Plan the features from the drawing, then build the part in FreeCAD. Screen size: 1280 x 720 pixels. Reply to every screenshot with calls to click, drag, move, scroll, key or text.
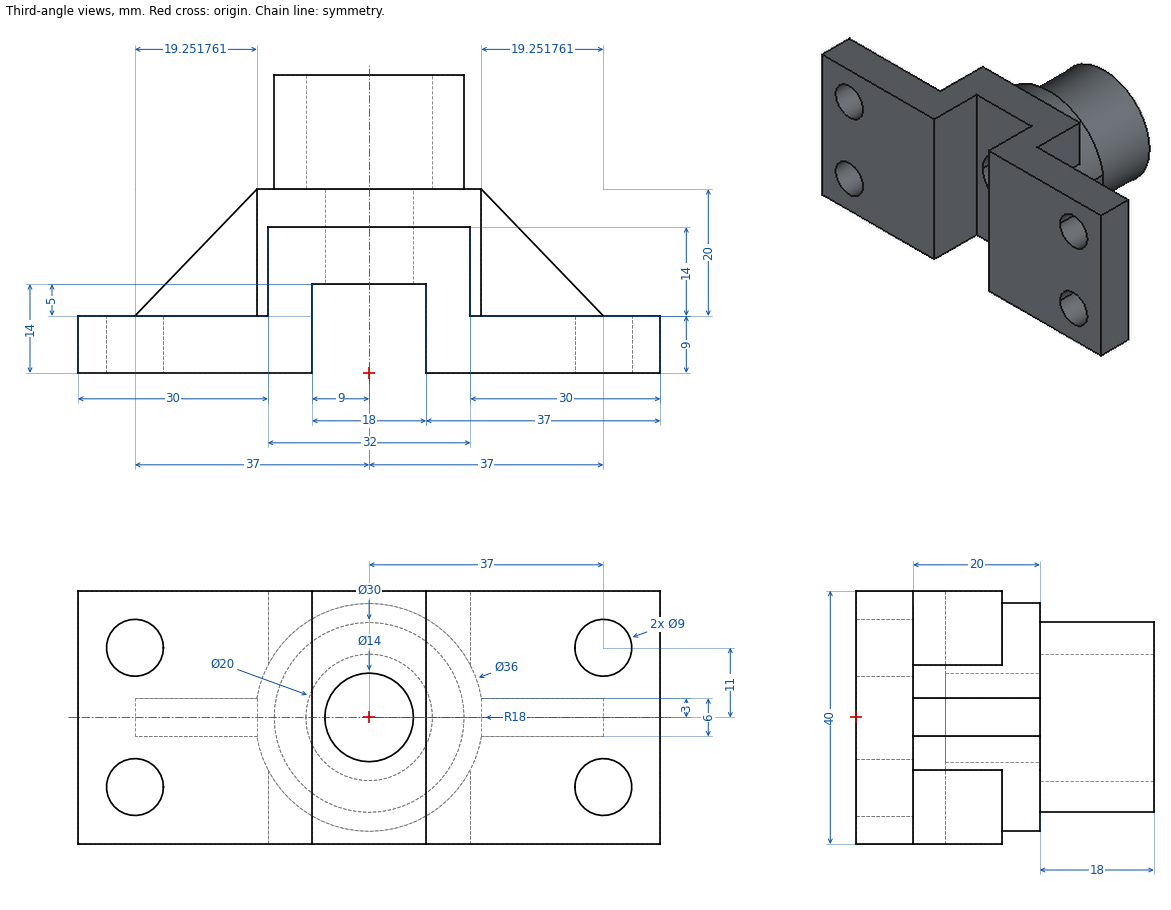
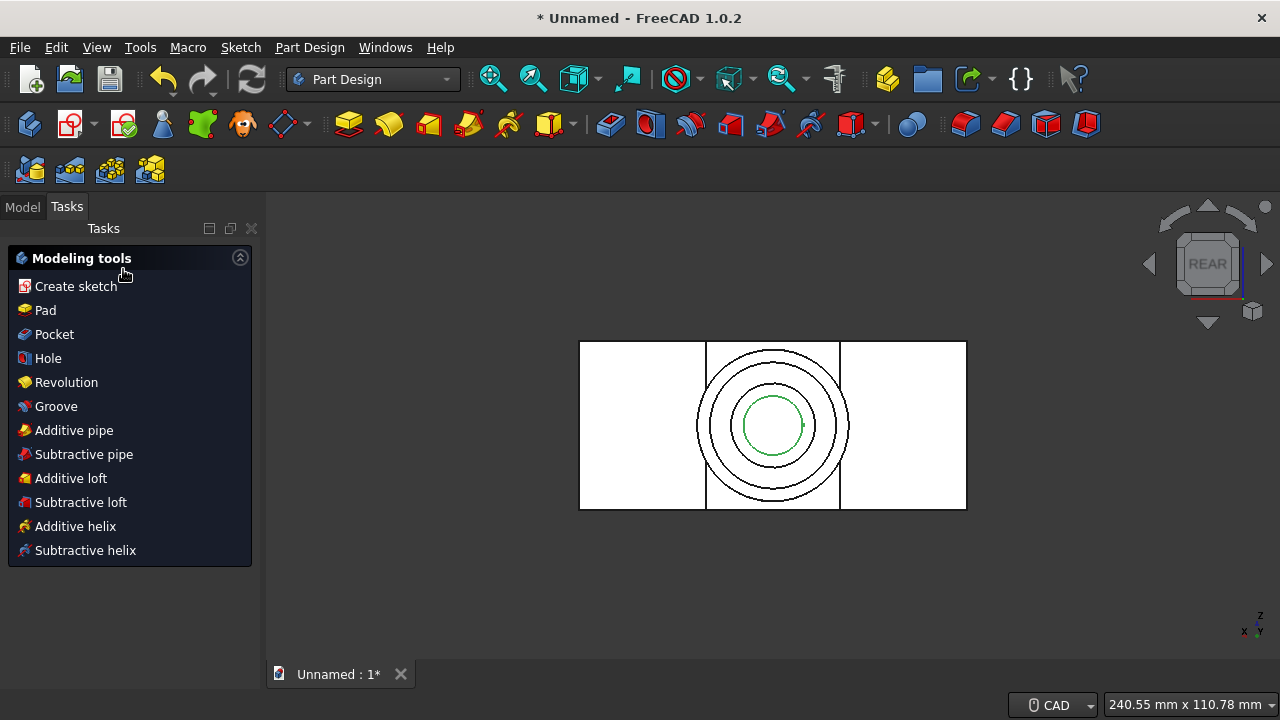
click(612, 124)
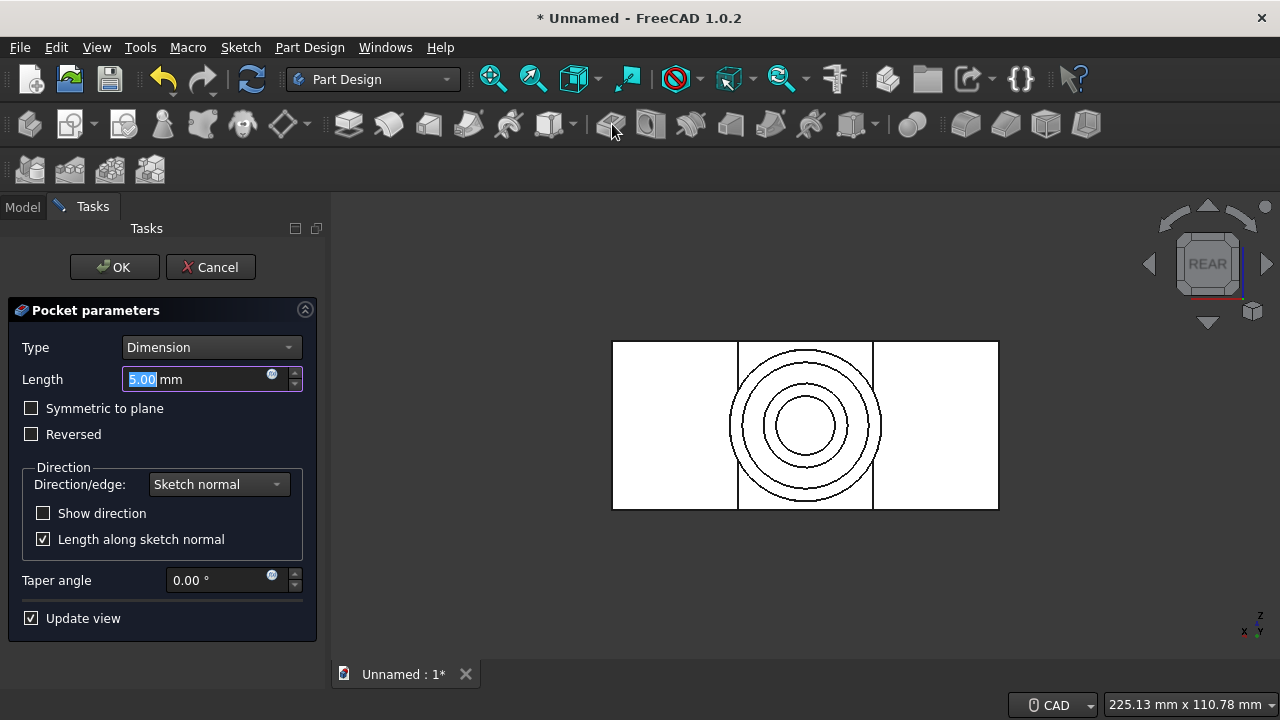
click(212, 348)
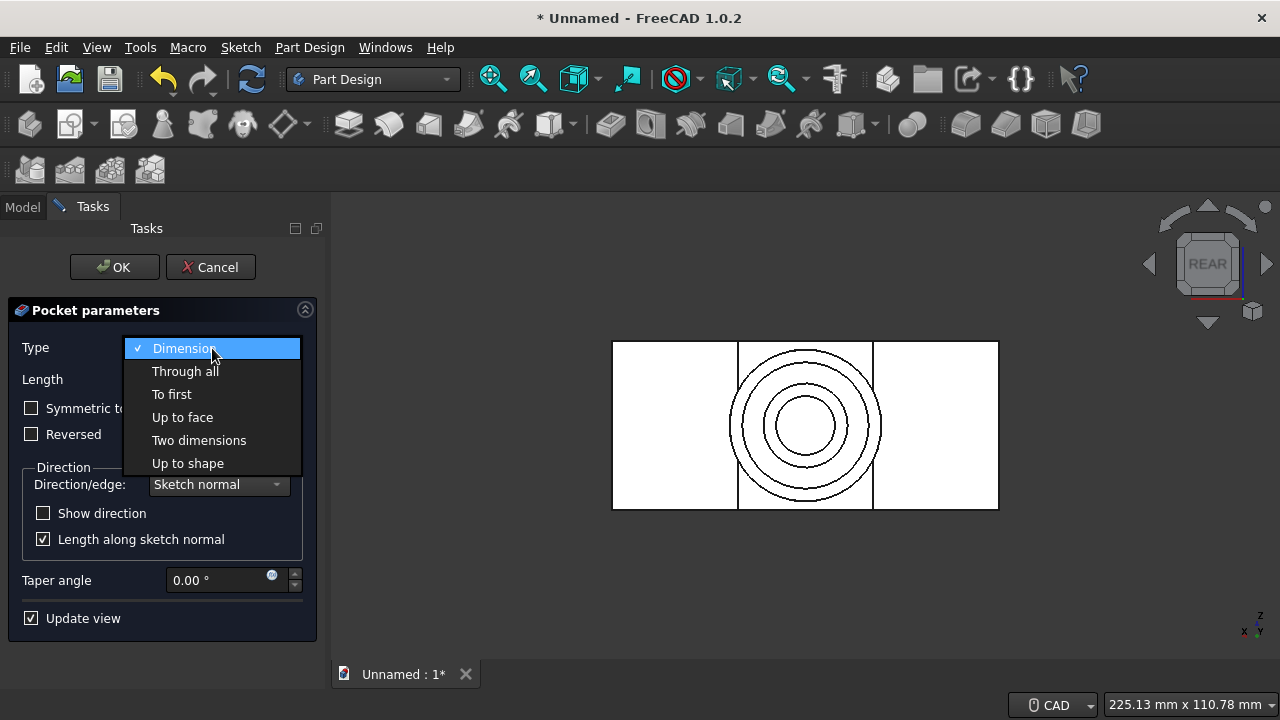
click(212, 372)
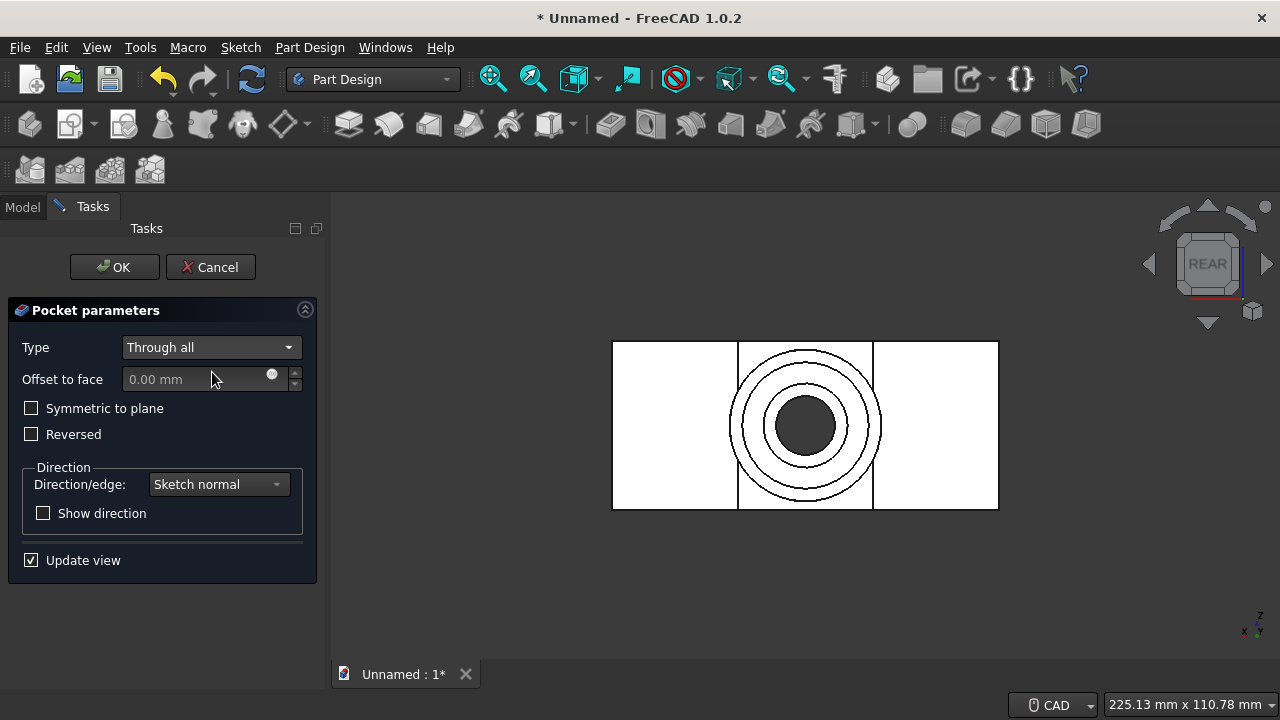
click(115, 267)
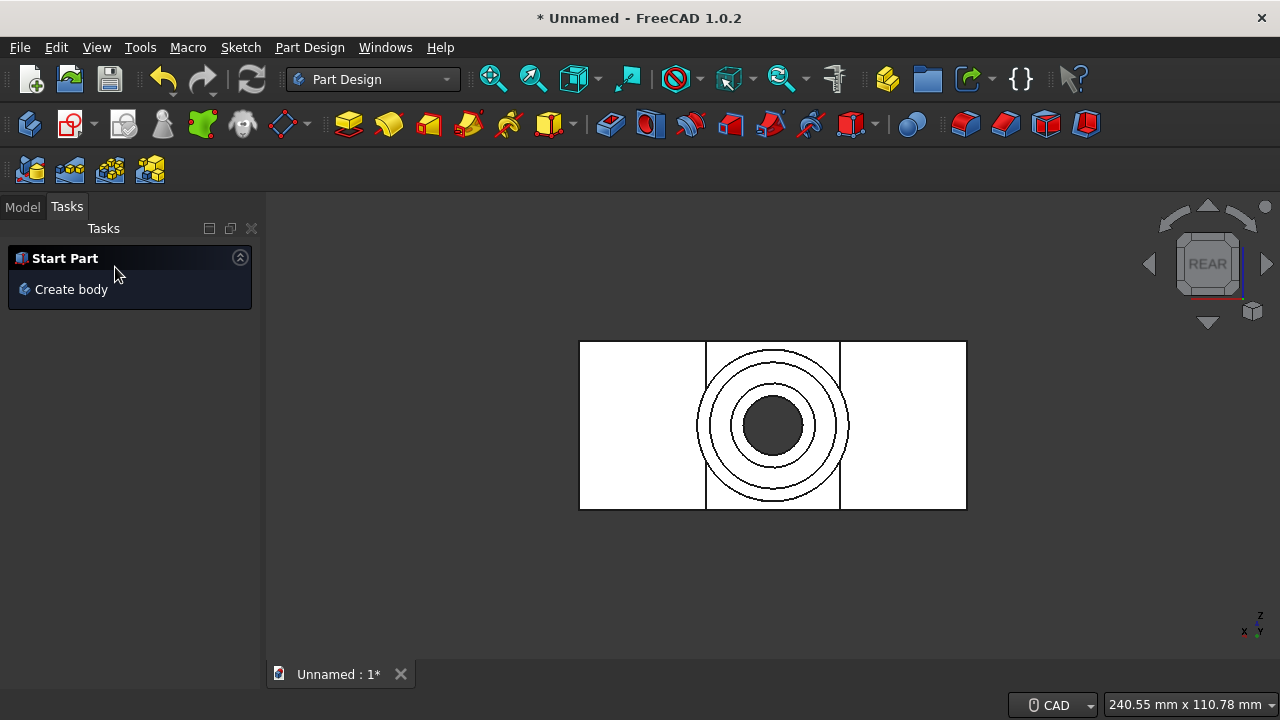
click(494, 80)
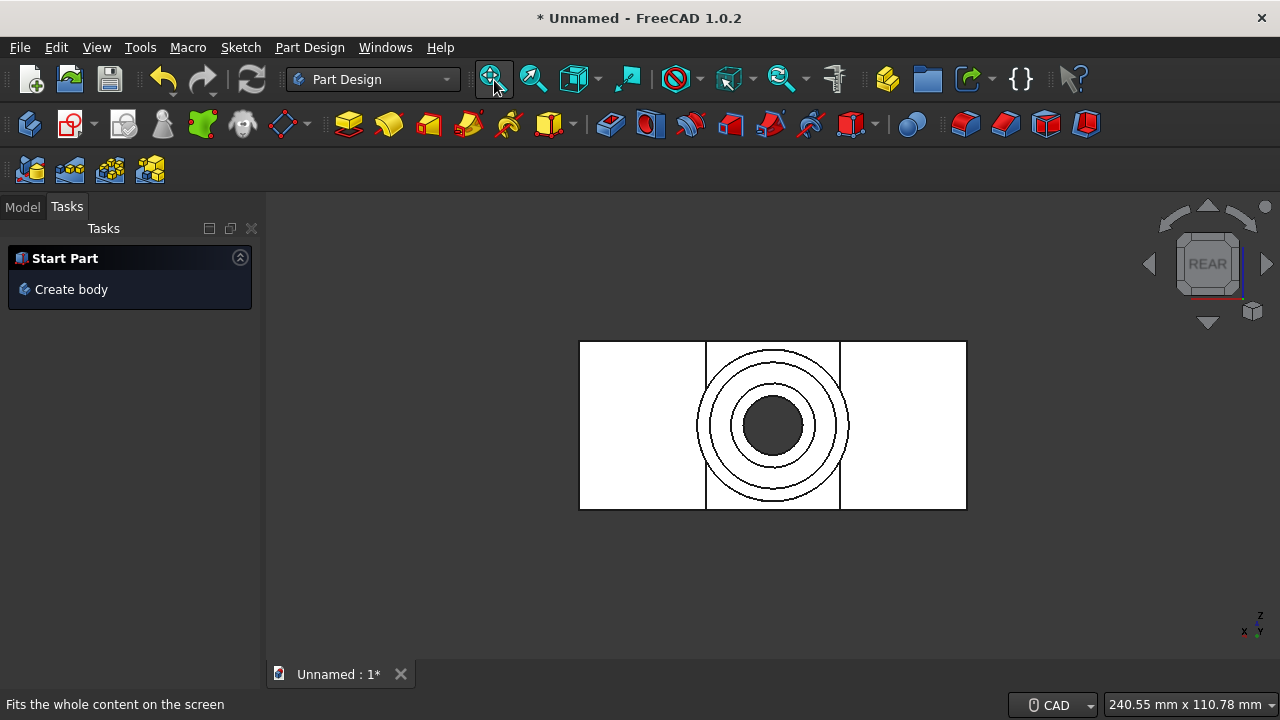
click(904, 400)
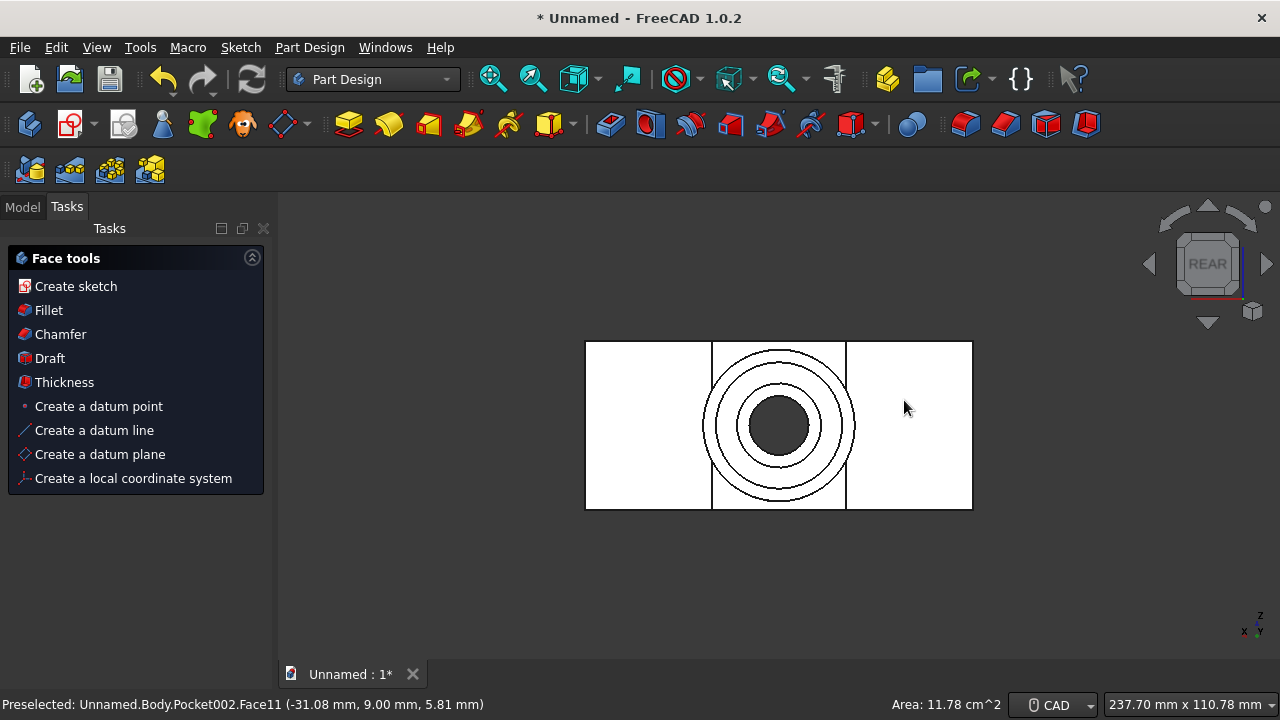
click(70, 124)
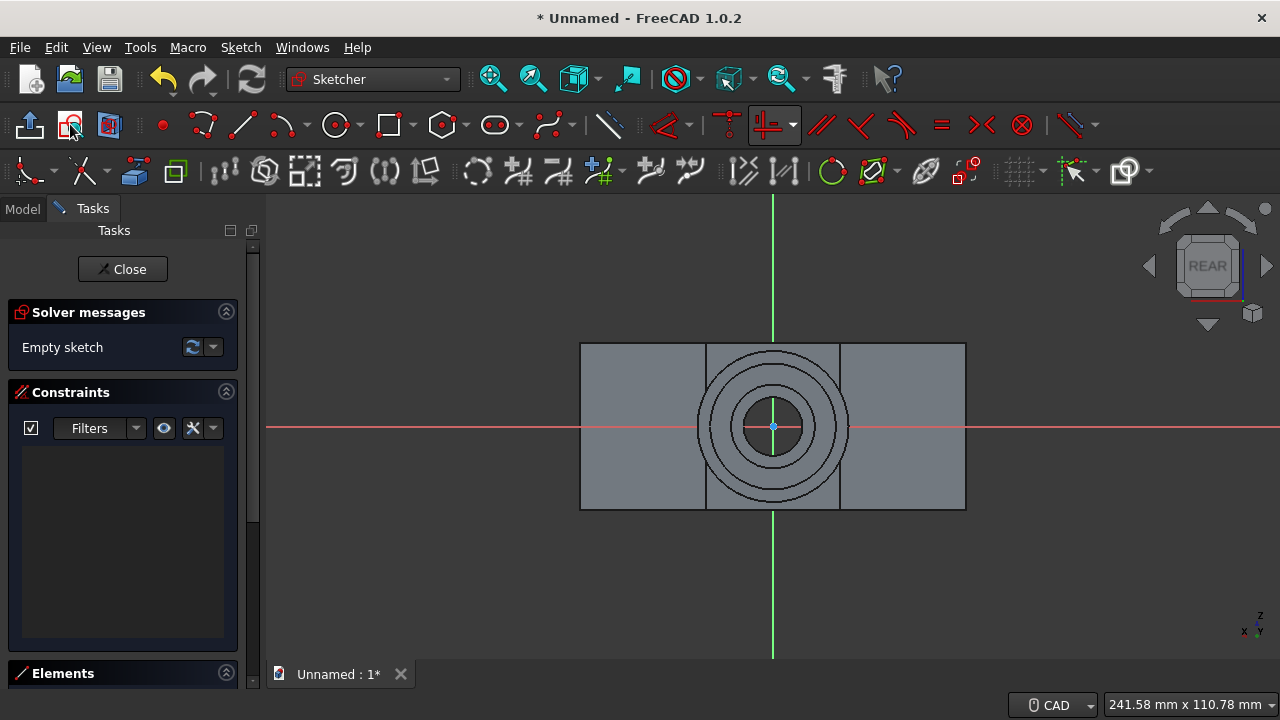
key(q)
key(s)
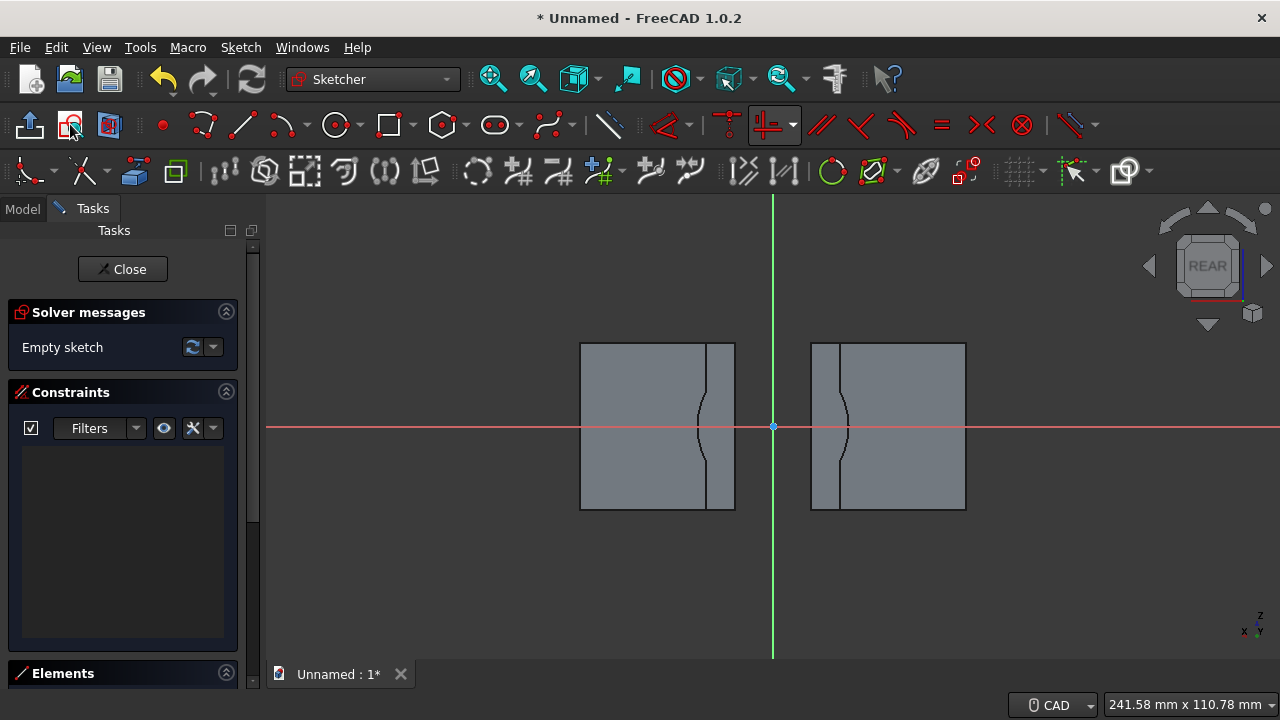
scroll(671, 426, up, 4)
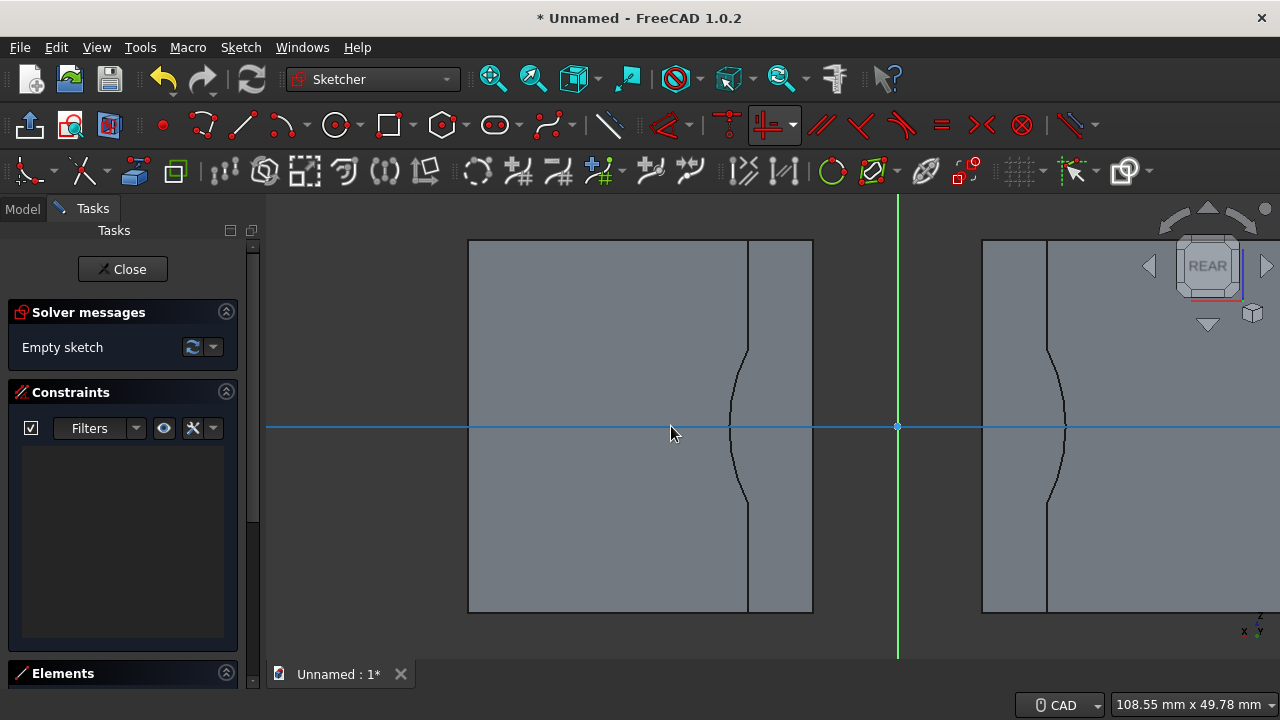
click(336, 126)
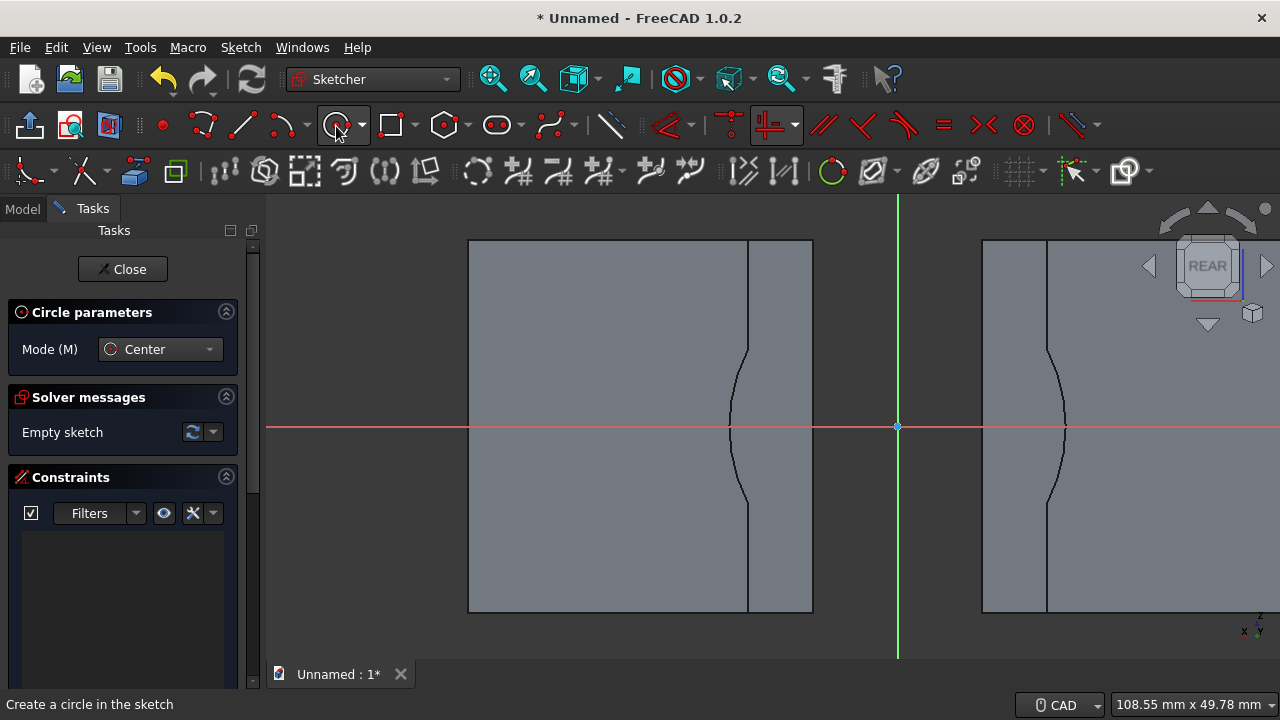
click(552, 324)
click(582, 294)